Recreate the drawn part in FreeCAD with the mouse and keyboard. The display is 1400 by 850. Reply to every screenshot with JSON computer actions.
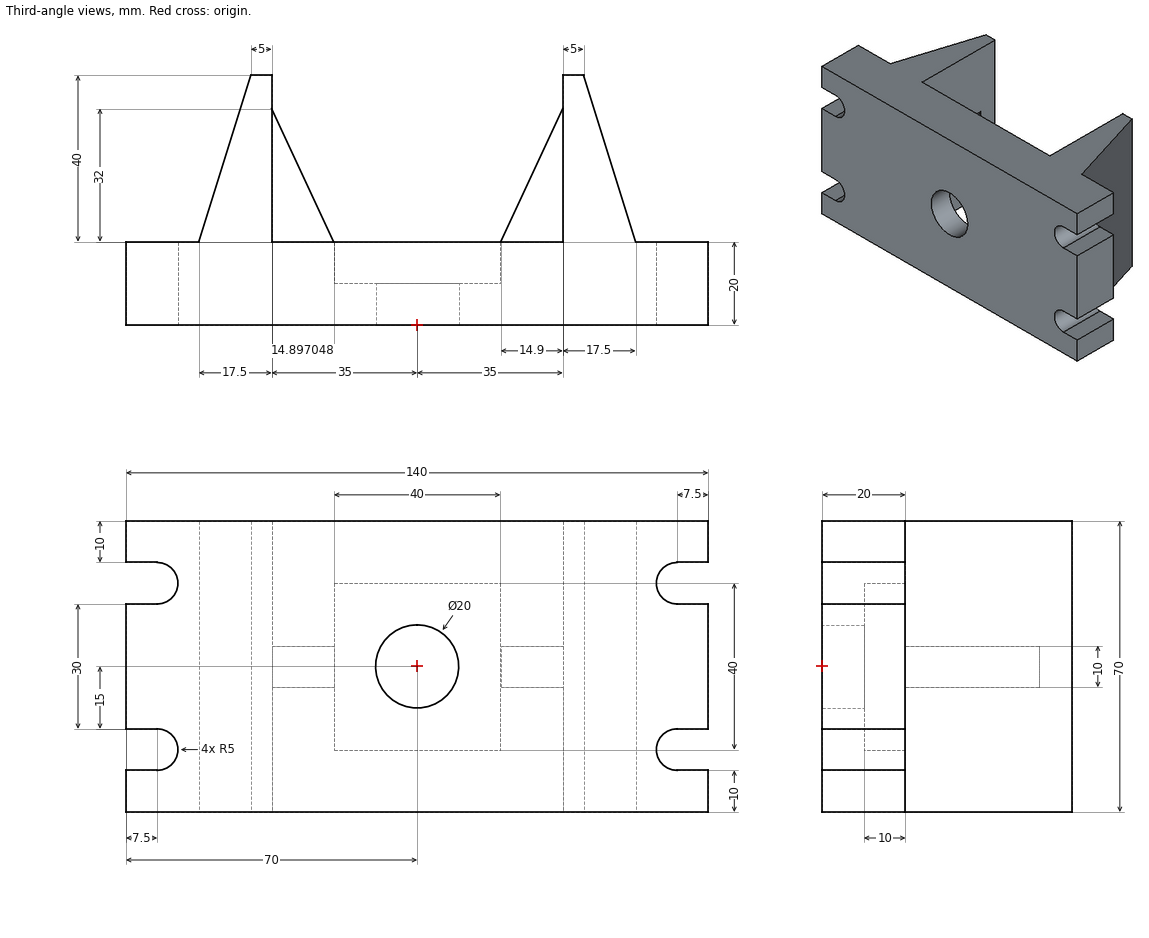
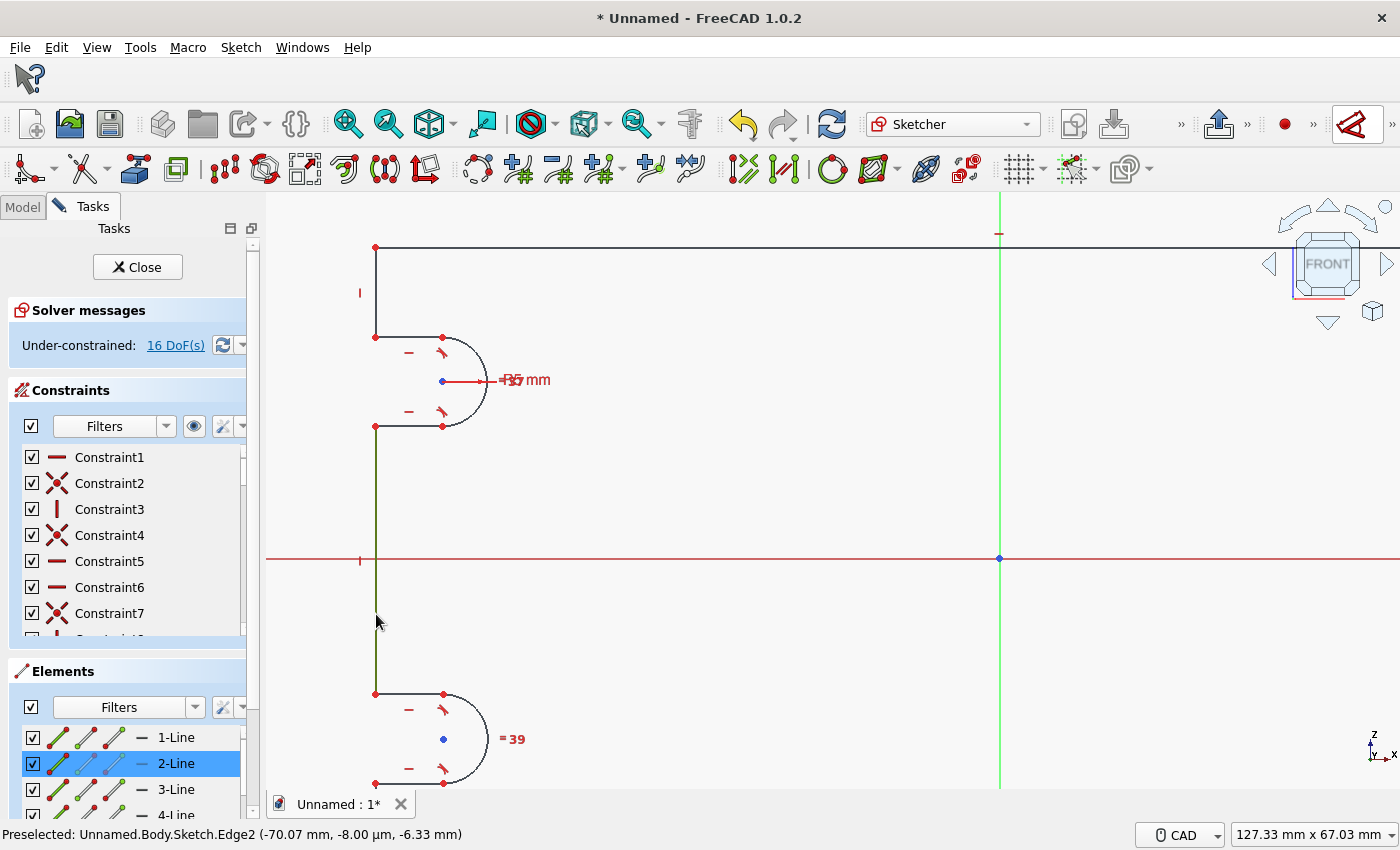
{"action": "left_click", "coordinate": [1378, 124]}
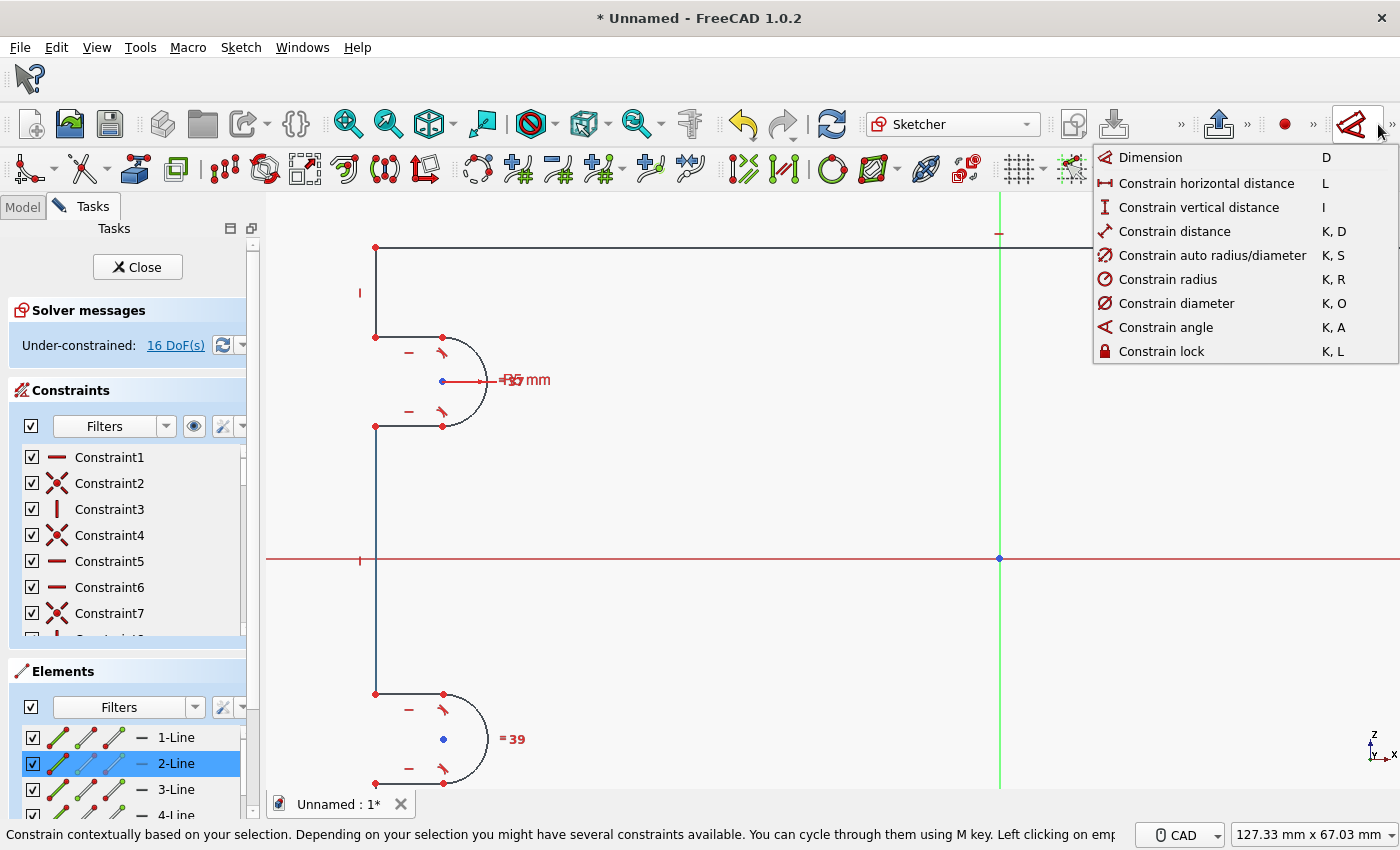
{"action": "left_click", "coordinate": [1246, 207]}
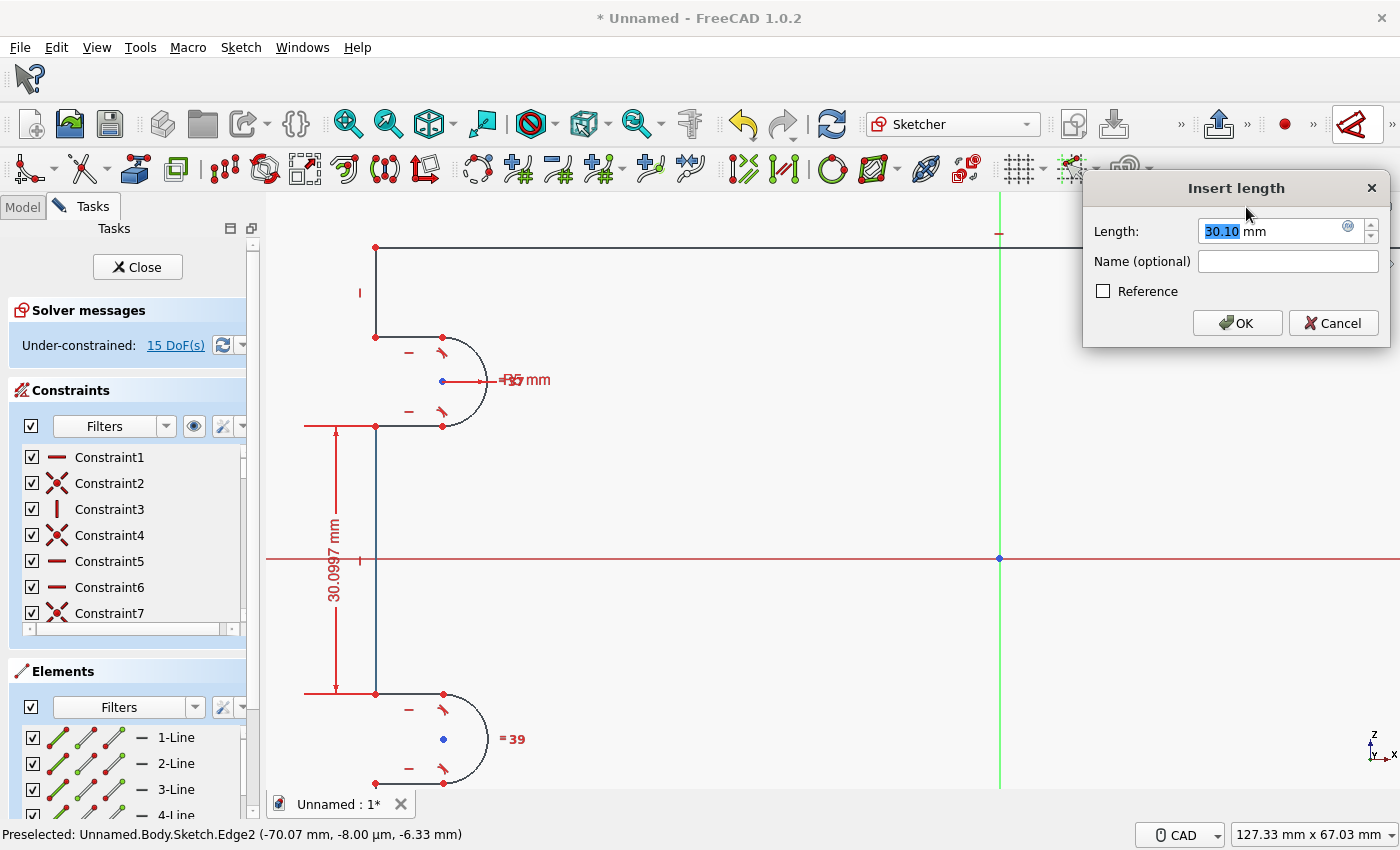
{"action": "type", "text": "30"}
{"action": "key", "text": "Return"}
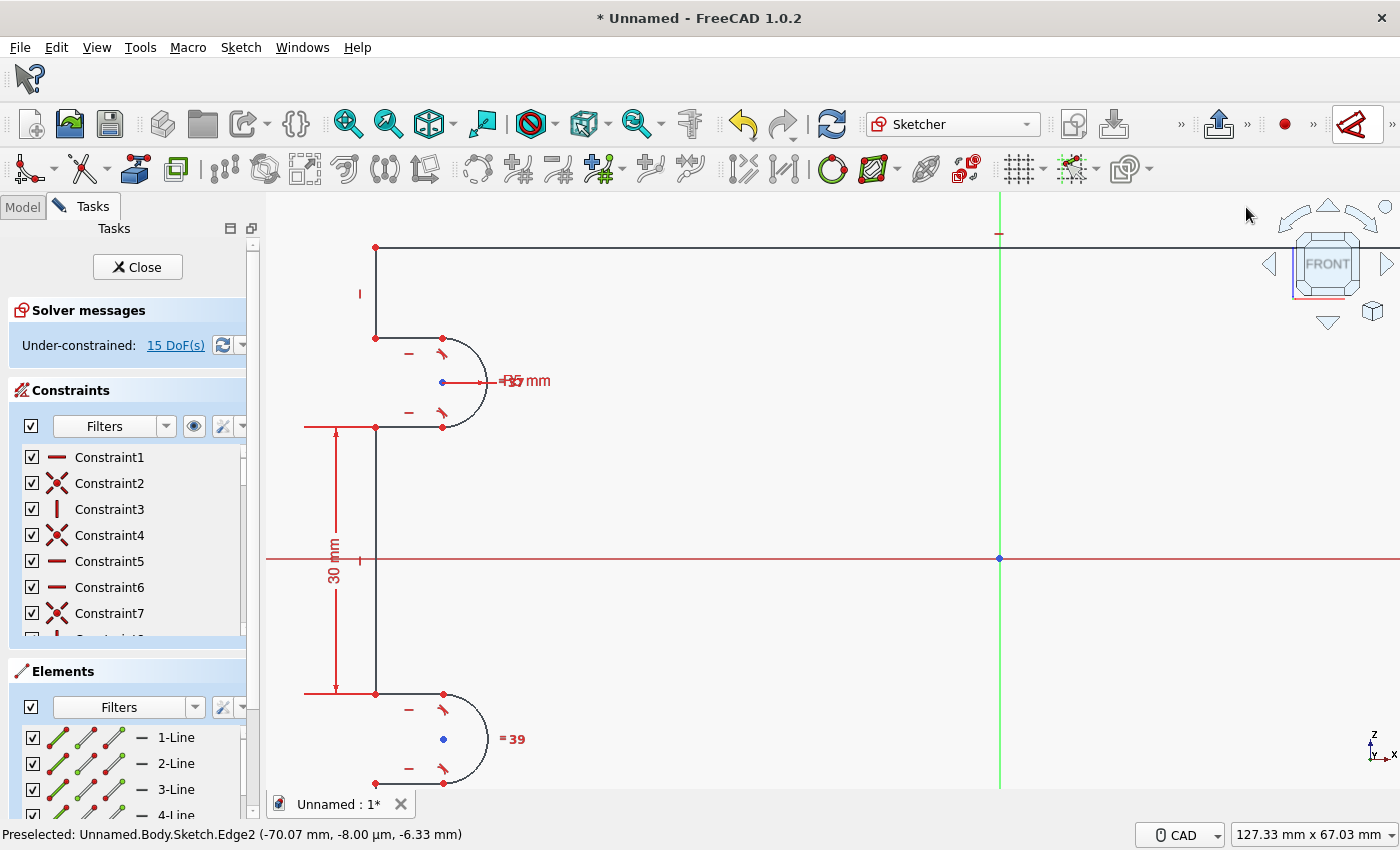
{"action": "left_click", "coordinate": [376, 311]}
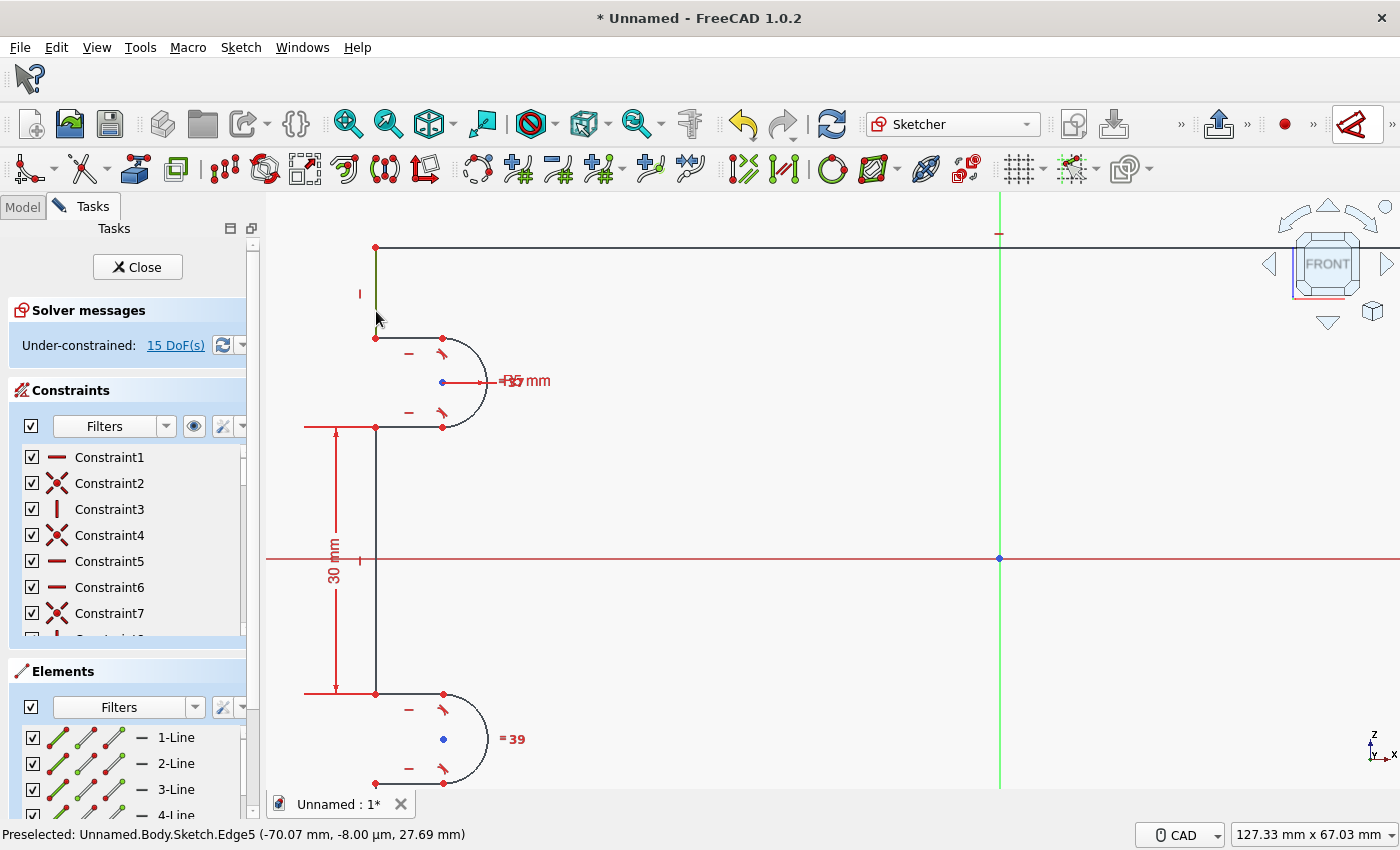
{"action": "left_click", "coordinate": [1378, 124]}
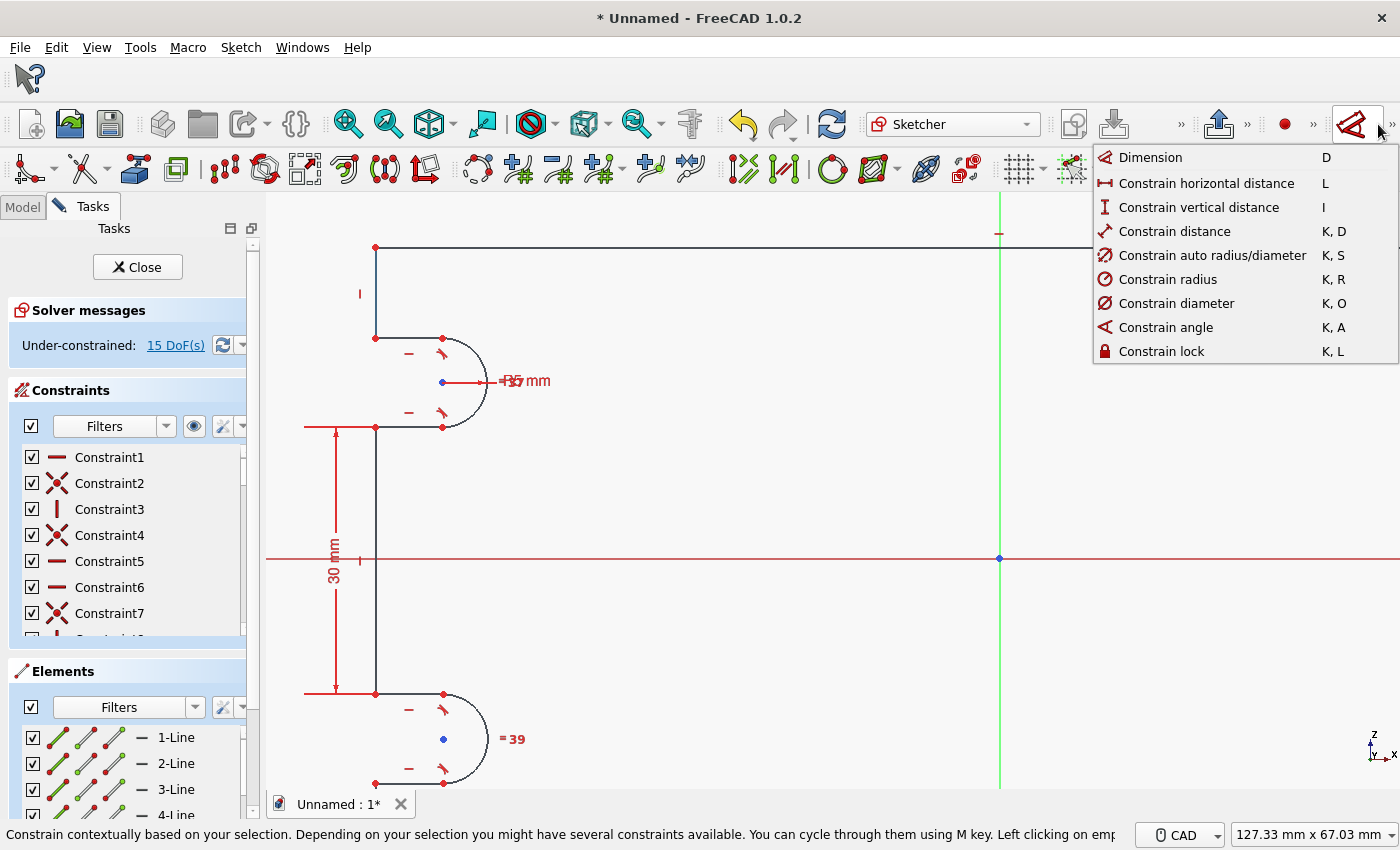
{"action": "left_click", "coordinate": [1246, 207]}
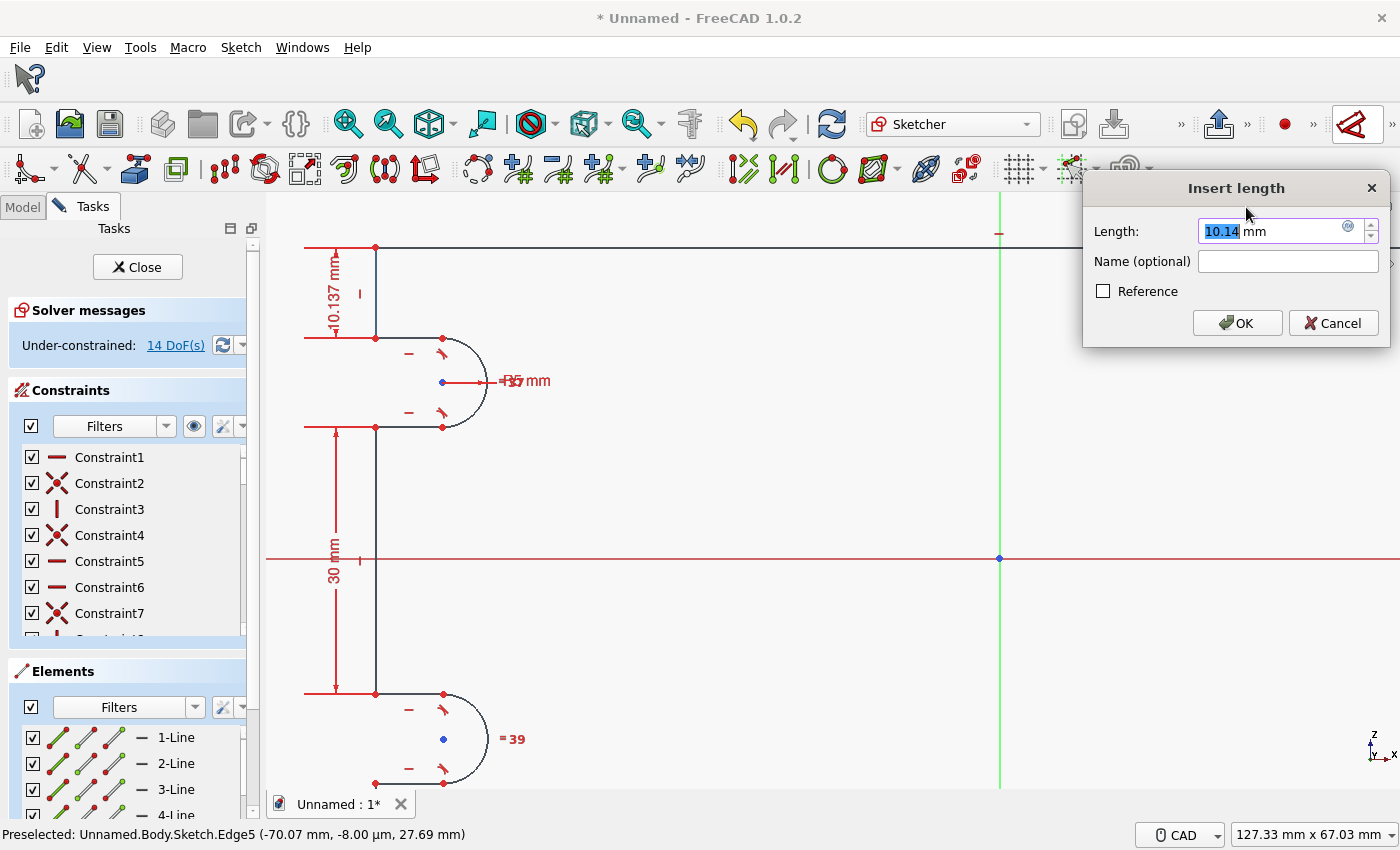
{"action": "type", "text": "10"}
{"action": "key", "text": "Return"}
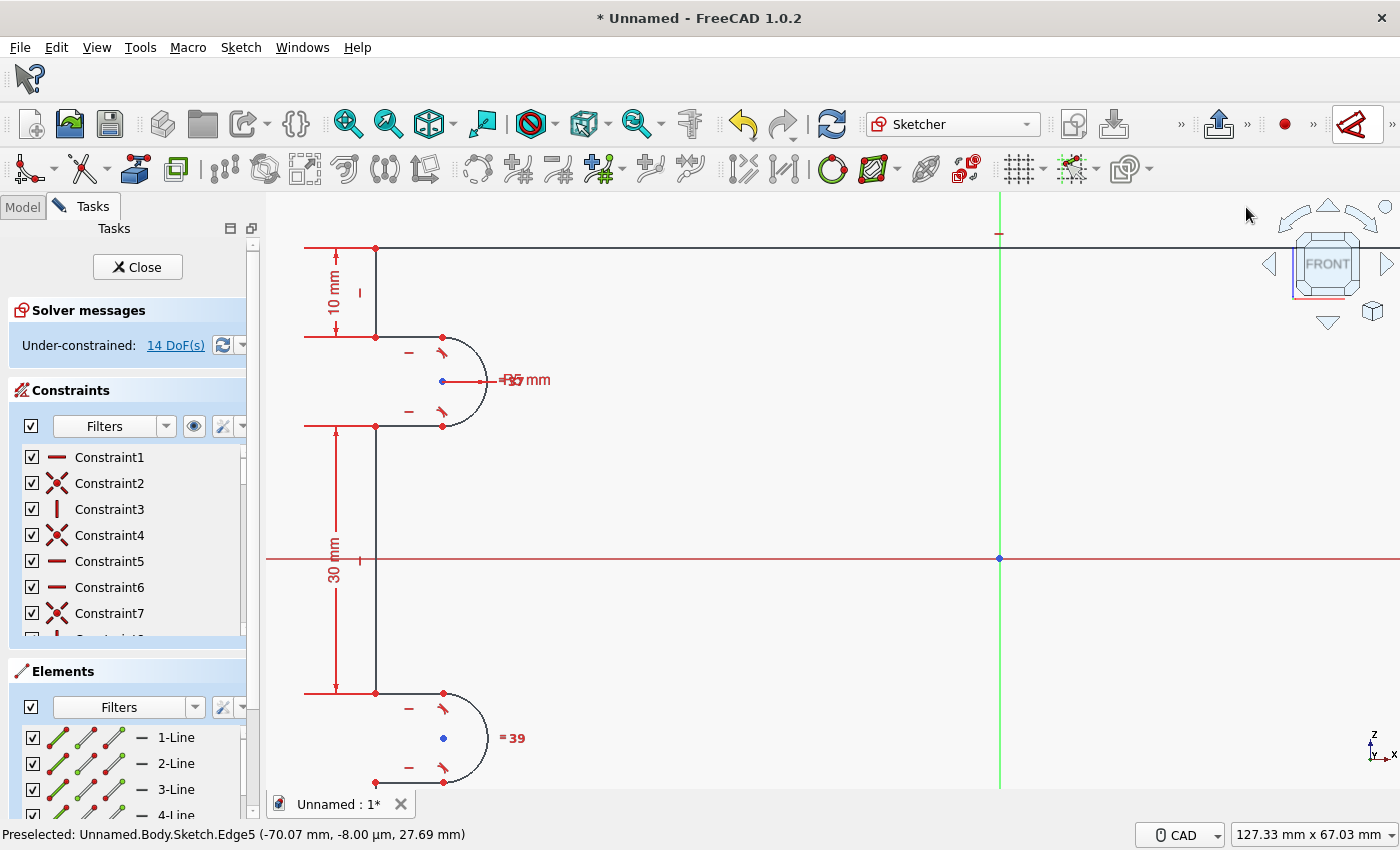
{"action": "scroll", "coordinate": [478, 408], "scroll_direction": "down", "scroll_amount": 3}